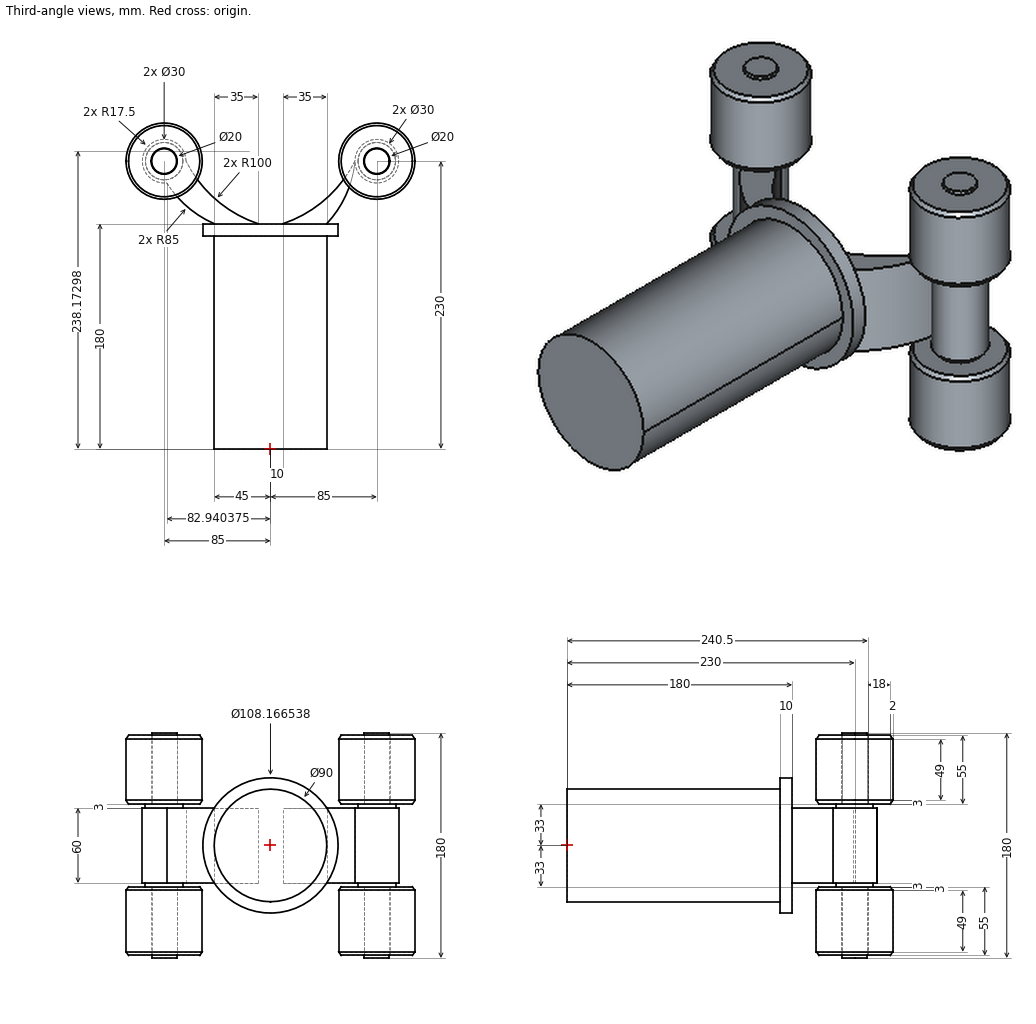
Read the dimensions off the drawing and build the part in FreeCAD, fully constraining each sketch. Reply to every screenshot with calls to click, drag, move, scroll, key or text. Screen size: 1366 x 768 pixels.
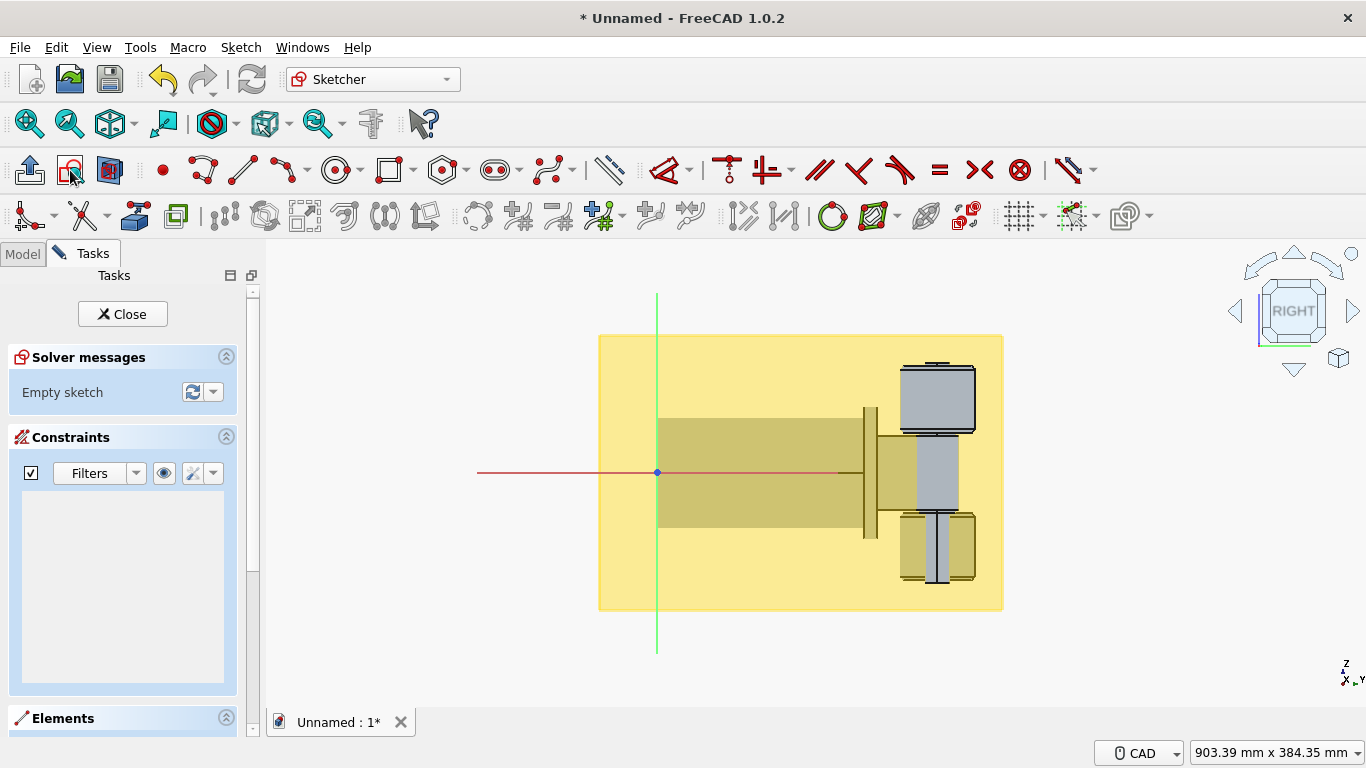
click(110, 170)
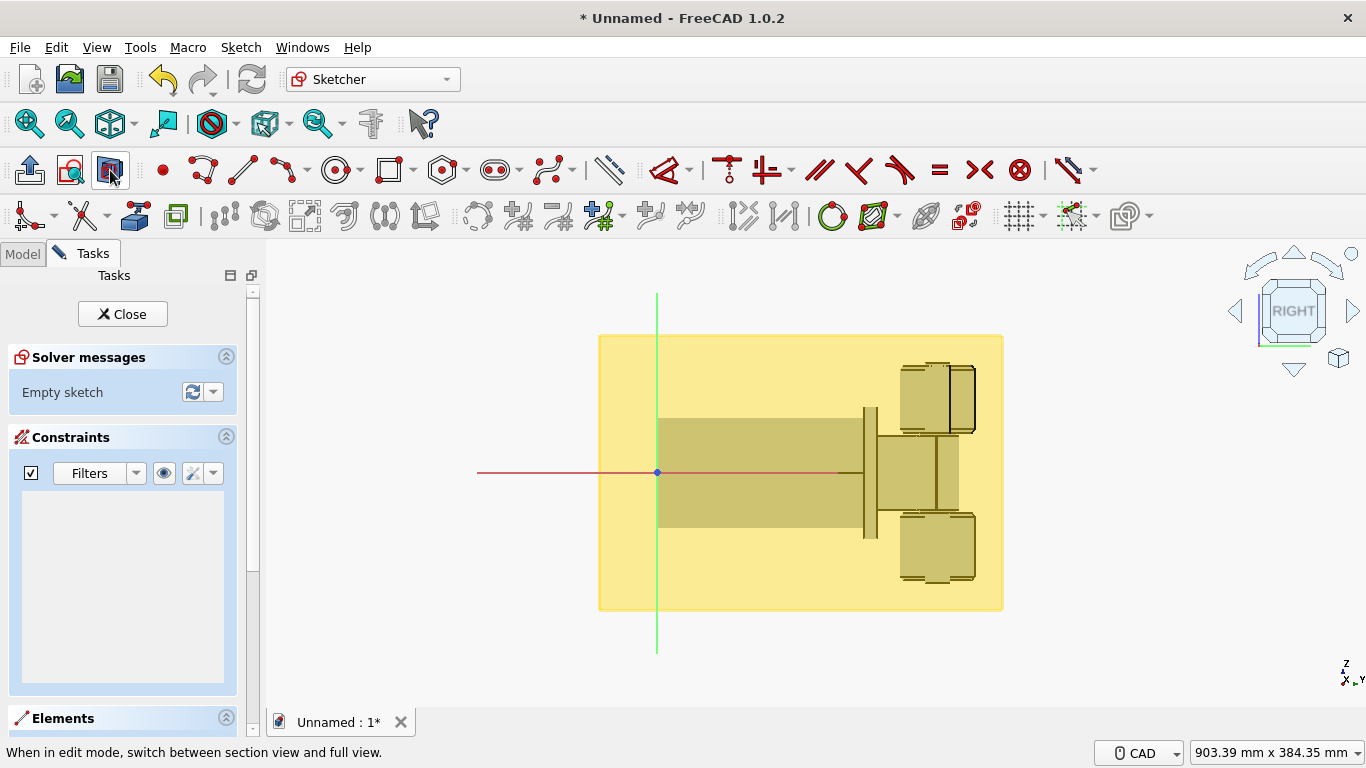
scroll(1046, 578, up, 6)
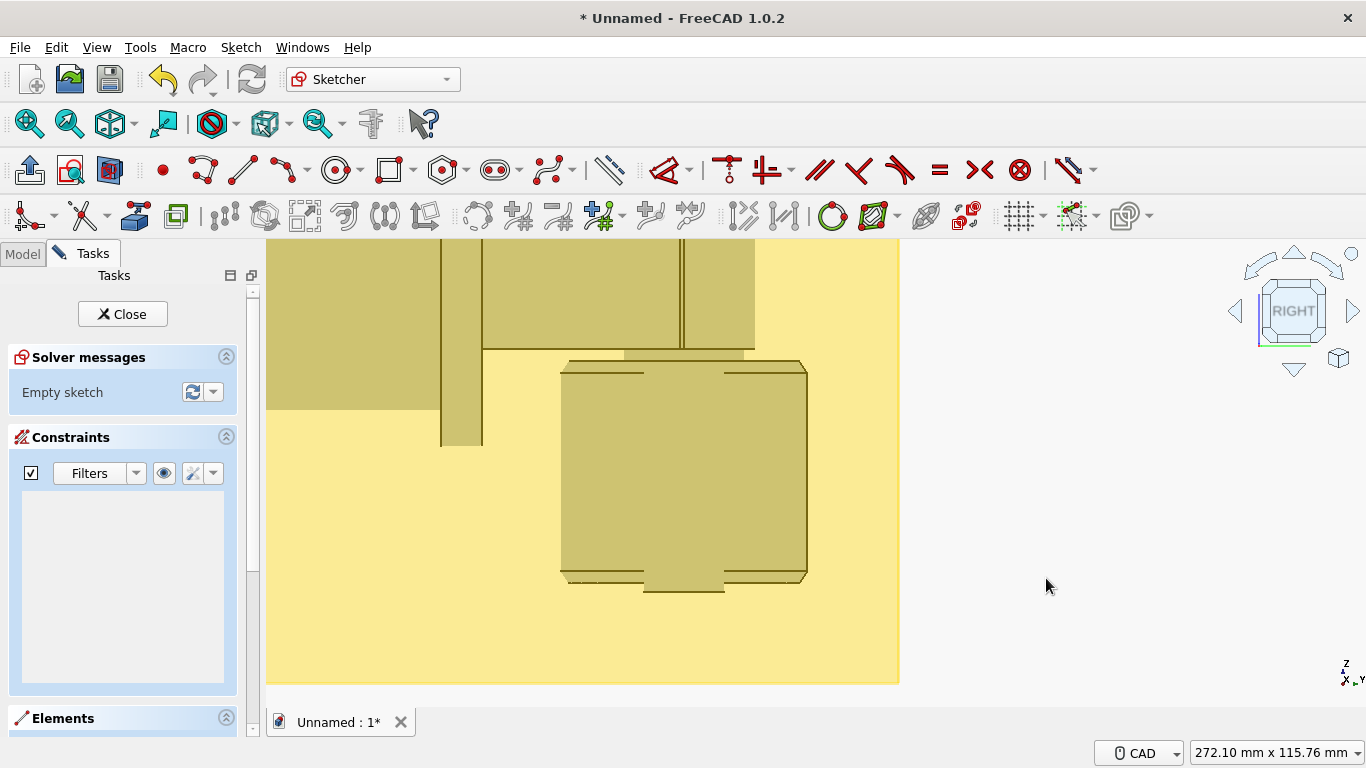
click(204, 170)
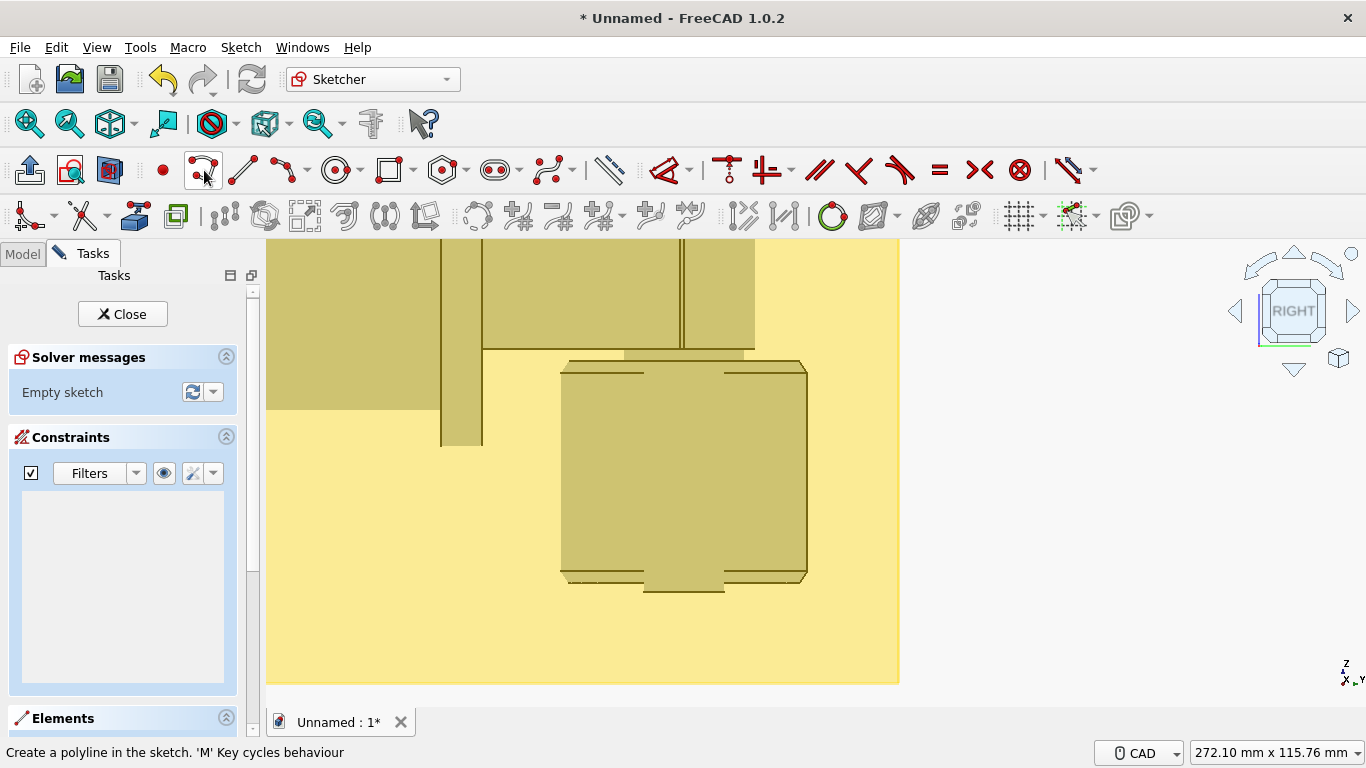
click(726, 361)
click(799, 361)
click(807, 373)
click(807, 571)
click(799, 583)
click(726, 583)
click(726, 362)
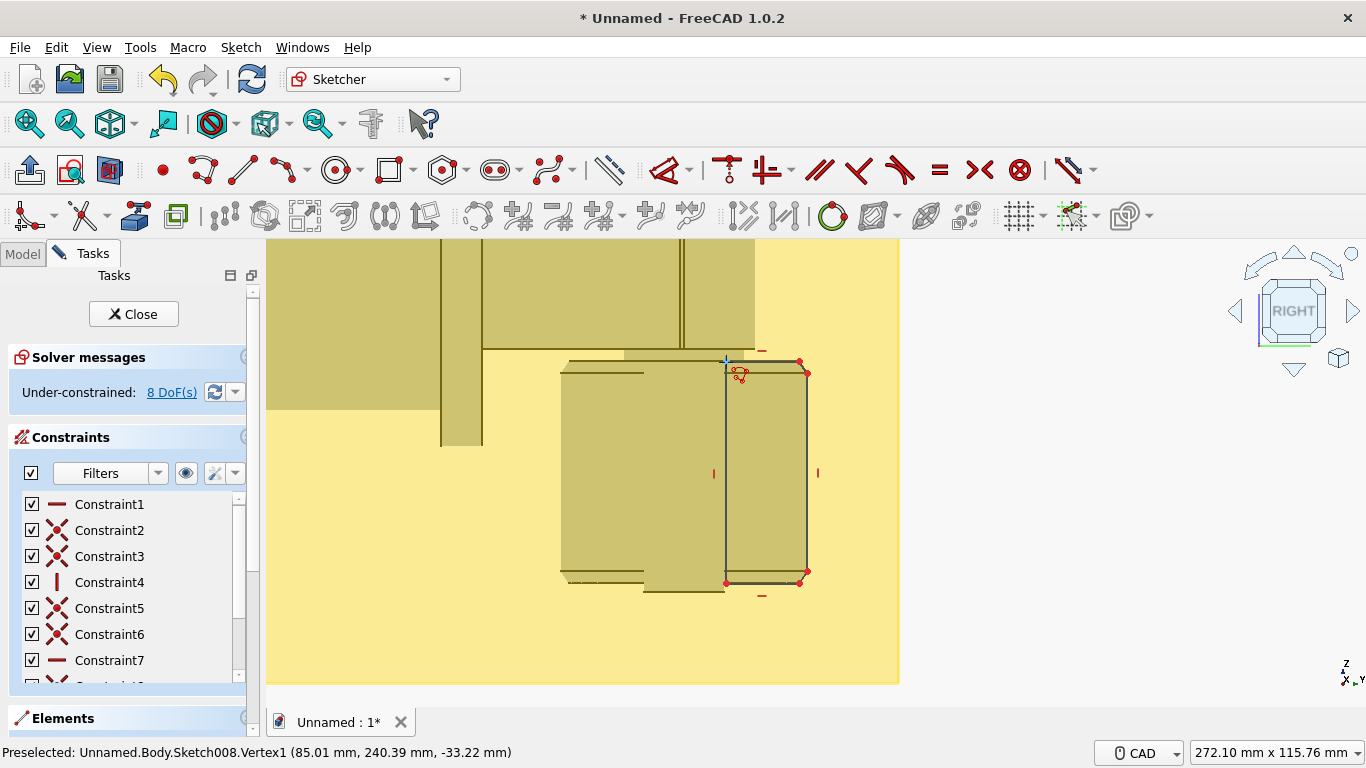
click(244, 170)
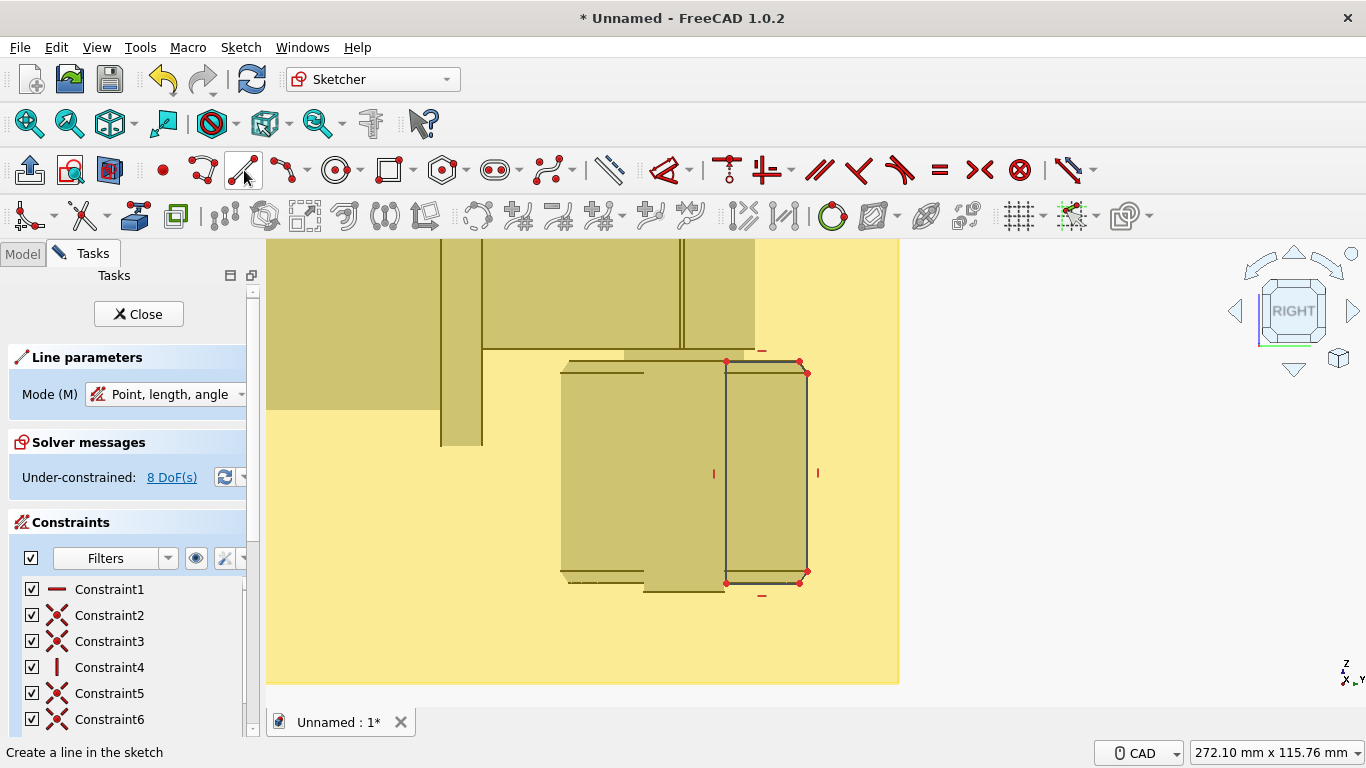
click(684, 339)
click(684, 606)
key(Escape)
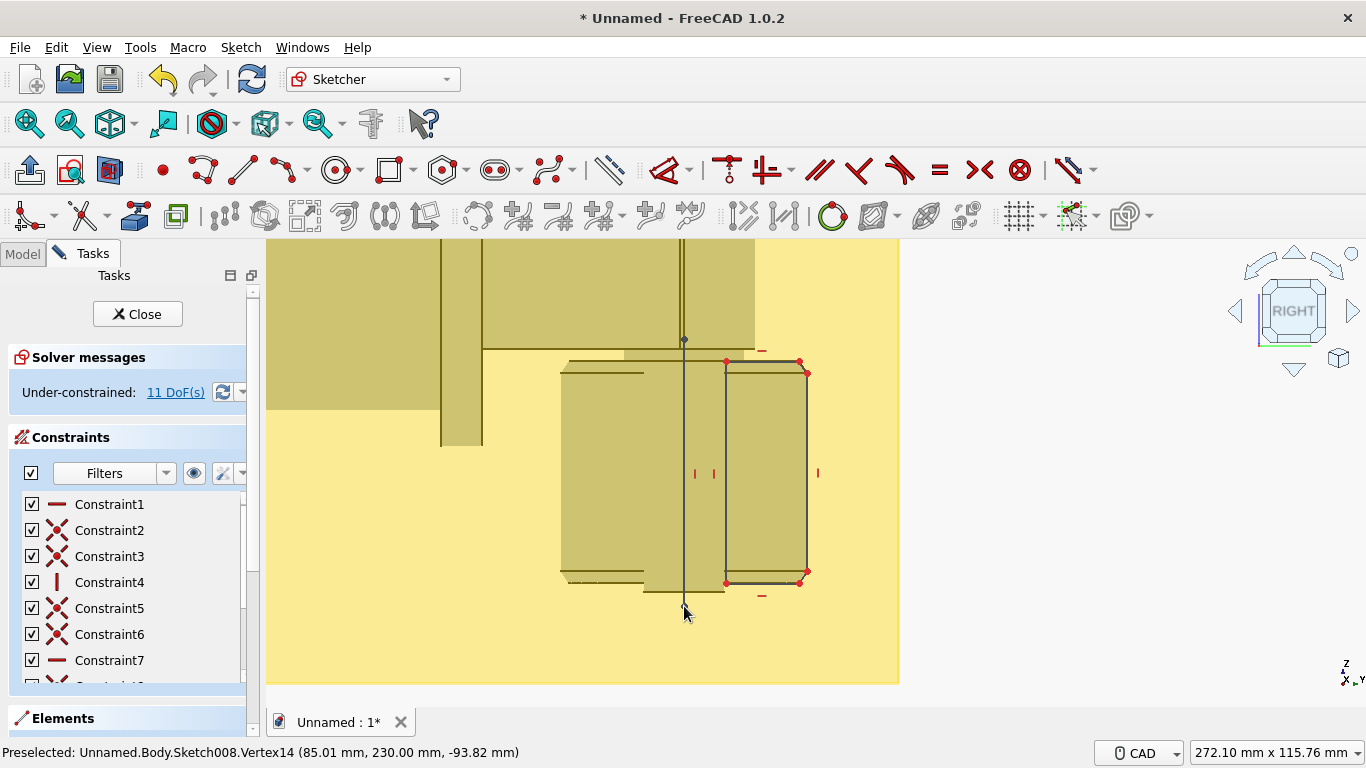
click(684, 420)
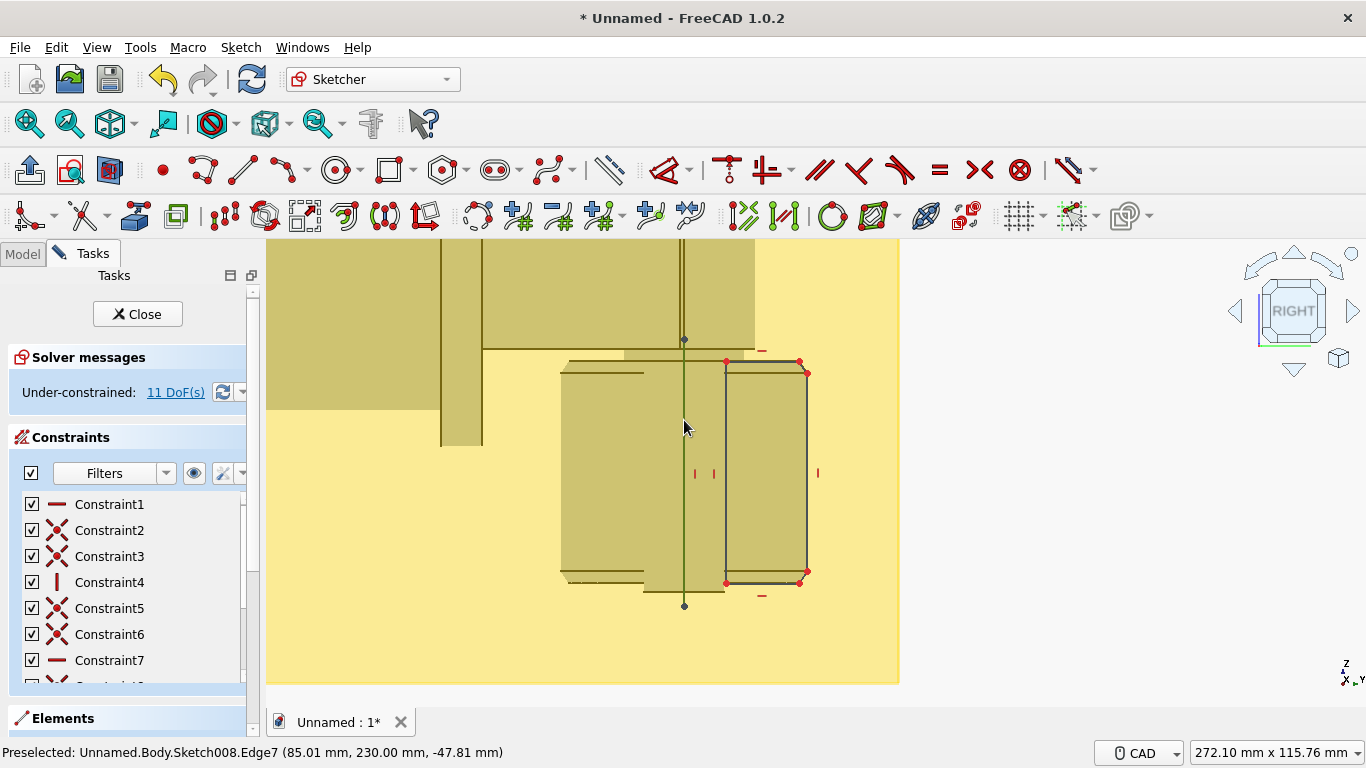
click(610, 170)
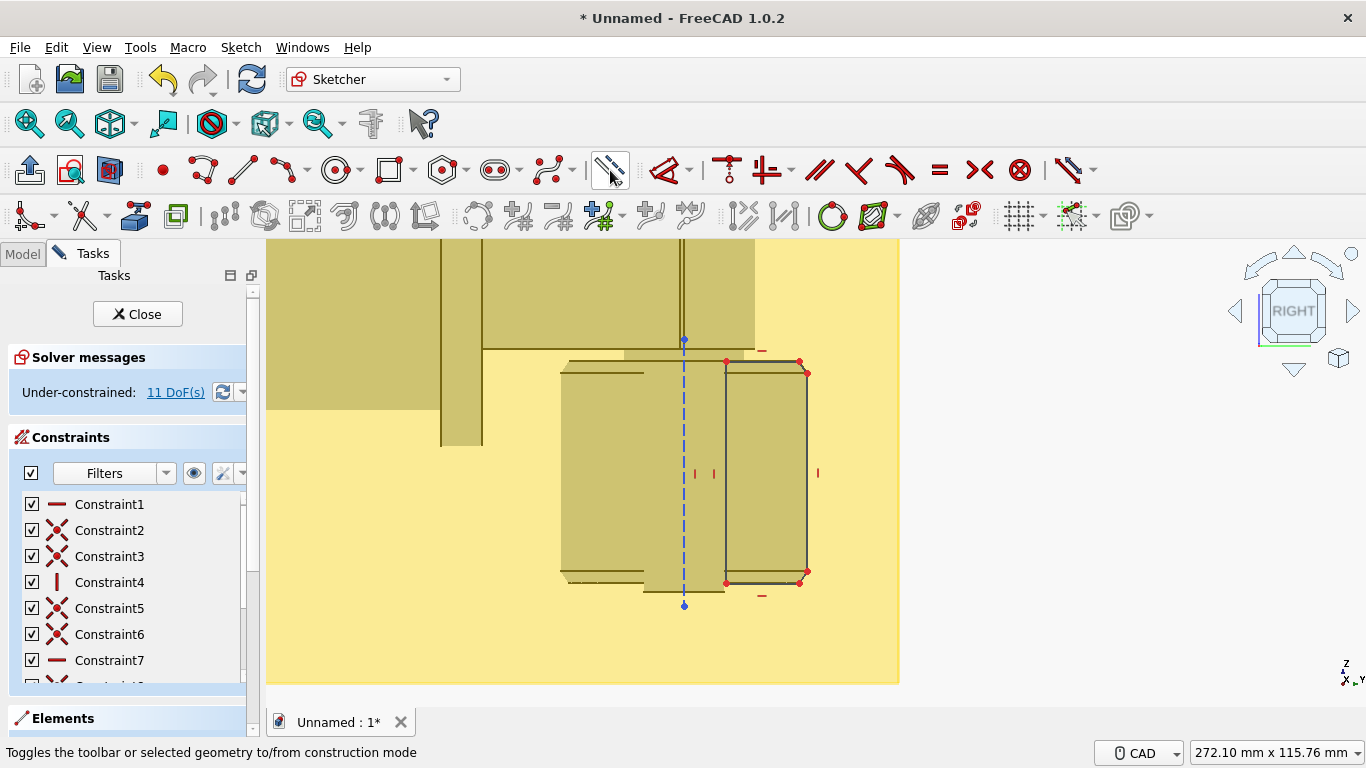
click(664, 170)